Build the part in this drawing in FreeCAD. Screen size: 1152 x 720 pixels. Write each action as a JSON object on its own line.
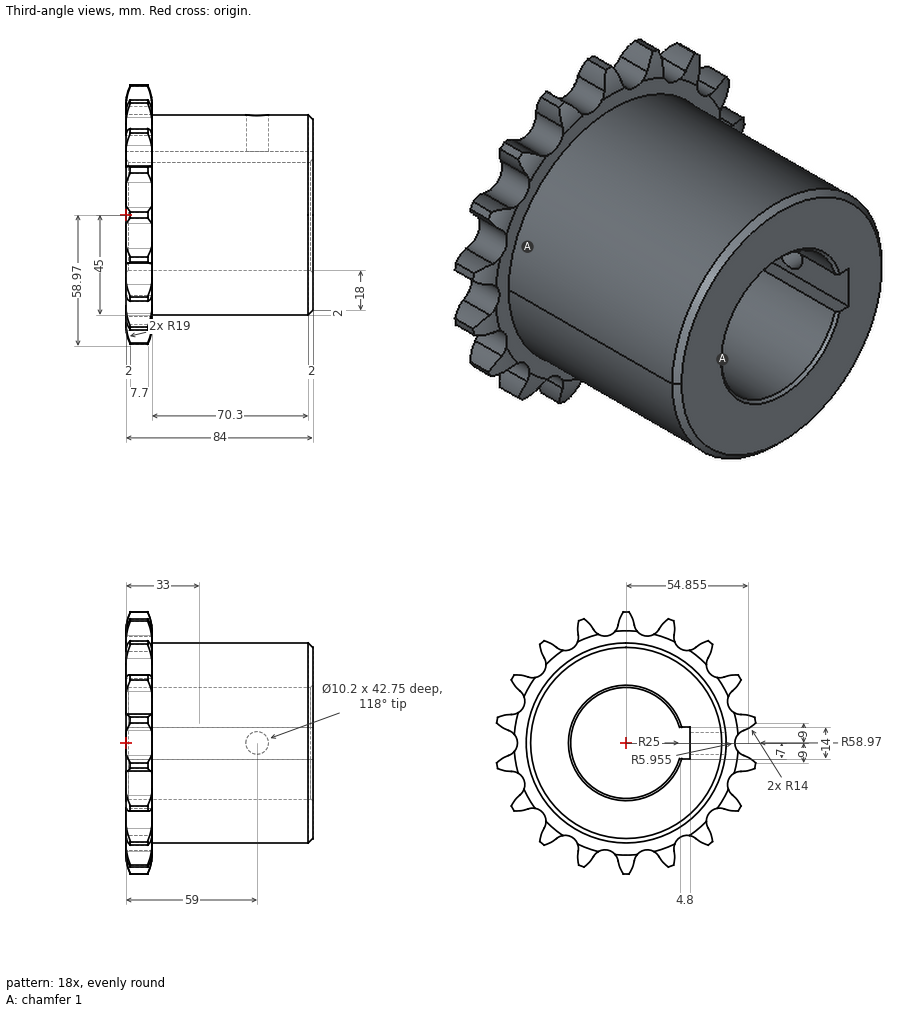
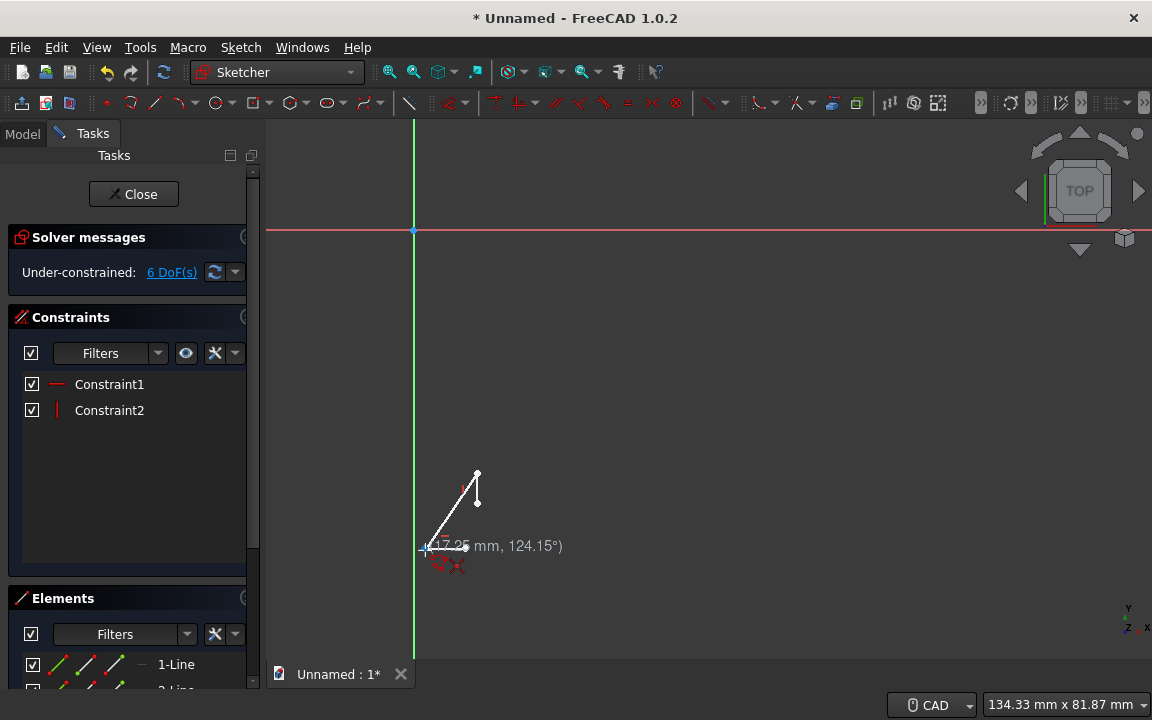
{"action": "left_click", "coordinate": [857, 473]}
{"action": "left_click", "coordinate": [868, 462]}
{"action": "left_click", "coordinate": [868, 365]}
{"action": "left_click", "coordinate": [414, 365]}
{"action": "left_click", "coordinate": [423, 503]}
{"action": "right_click", "coordinate": [423, 503]}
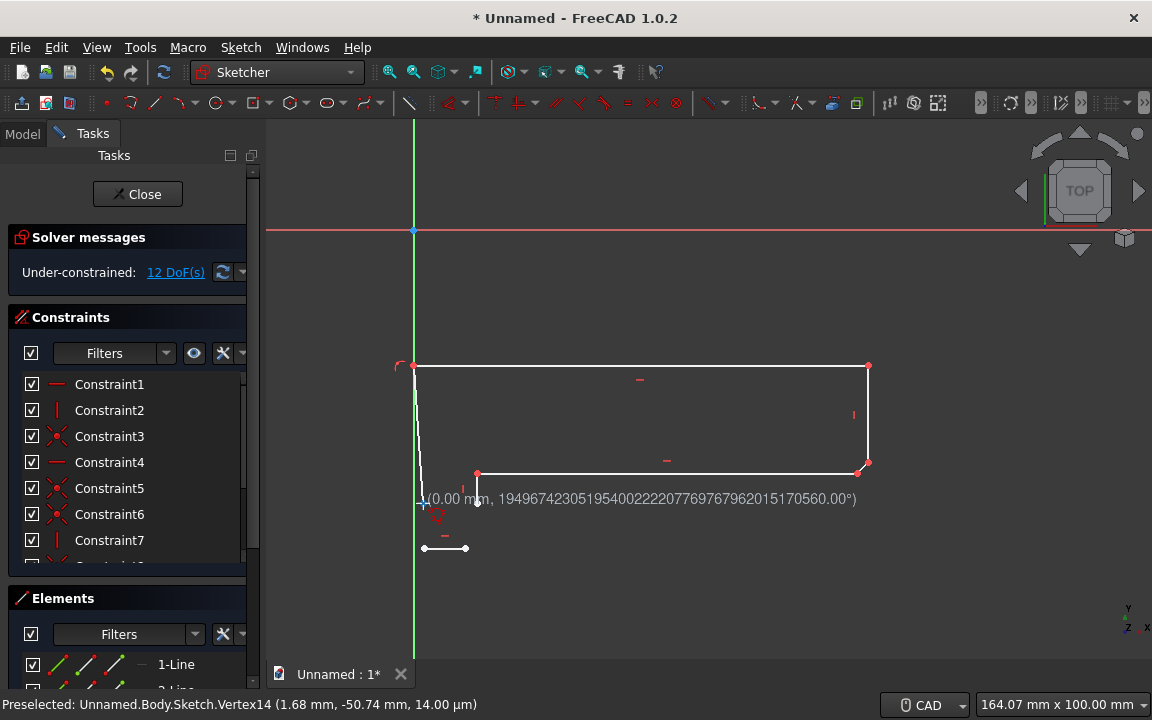
{"action": "key", "text": "g 3 a"}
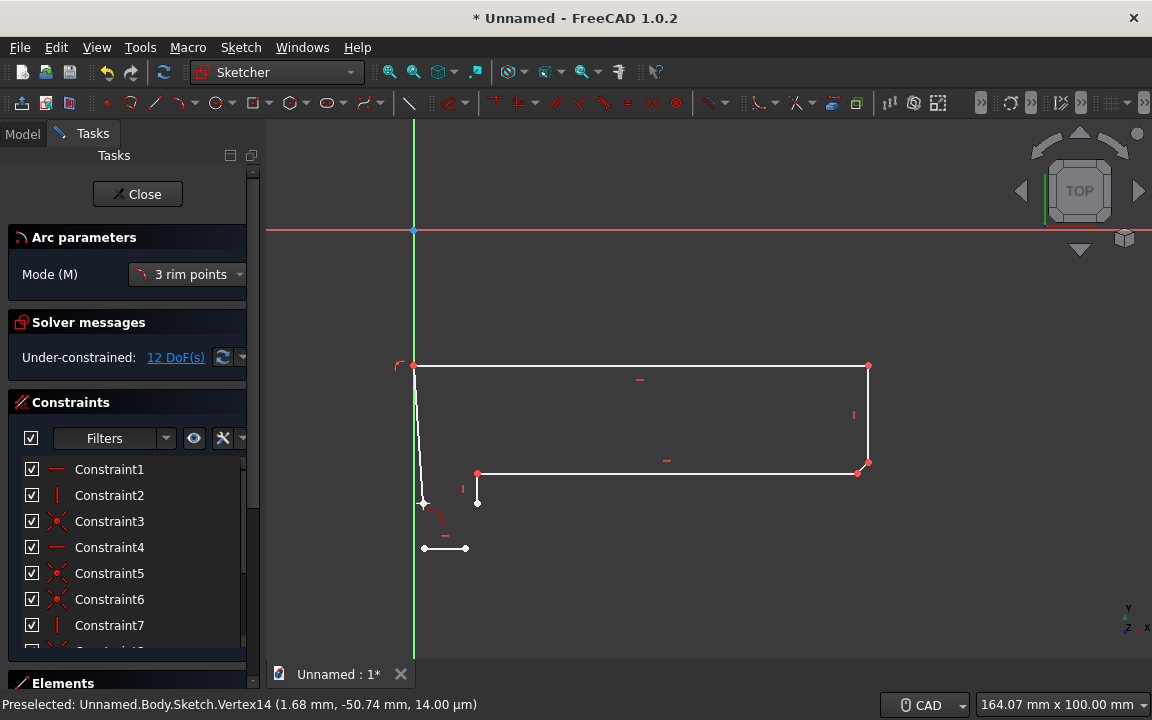
{"action": "left_click", "coordinate": [466, 549]}
{"action": "left_click", "coordinate": [477, 503]}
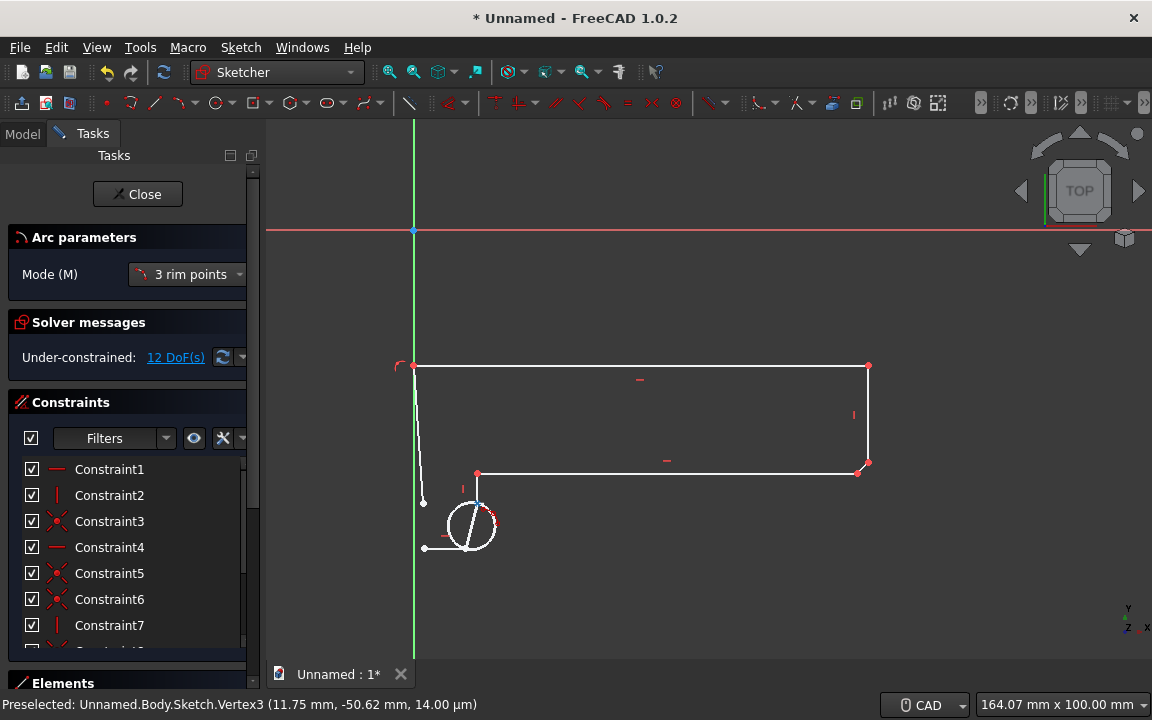
{"action": "scroll", "coordinate": [474, 526], "scroll_direction": "up", "scroll_amount": 9}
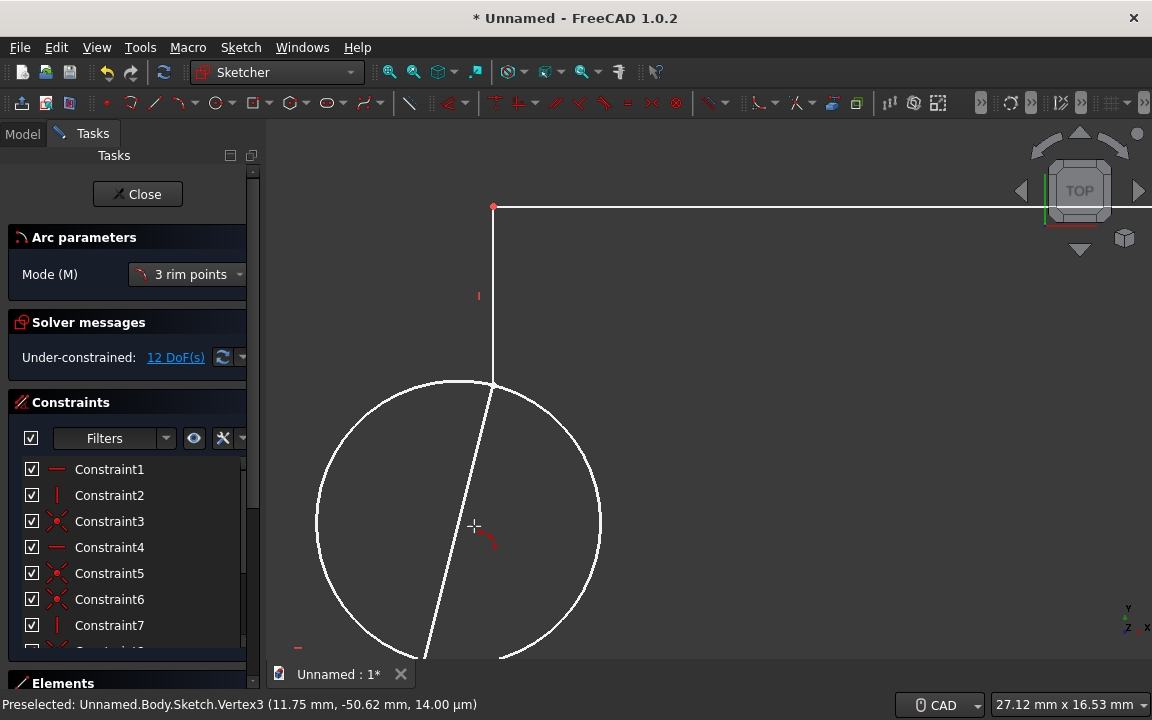
{"action": "left_click", "coordinate": [475, 523]}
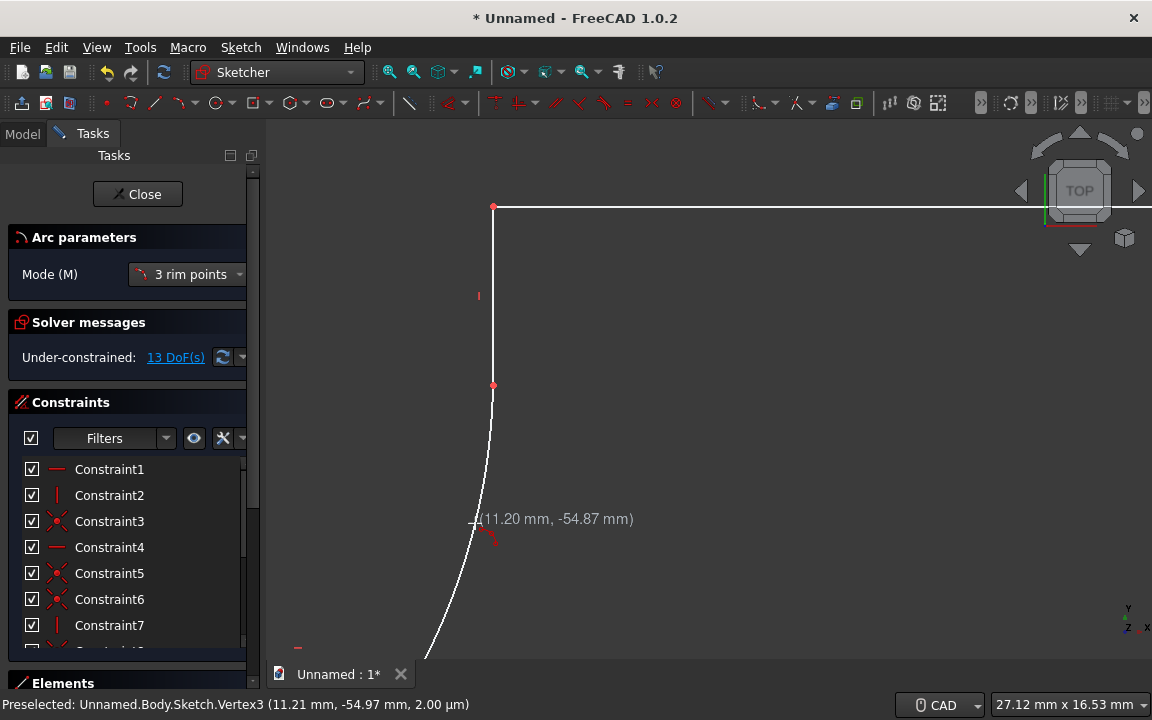
{"action": "scroll", "coordinate": [474, 526], "scroll_direction": "down", "scroll_amount": 9}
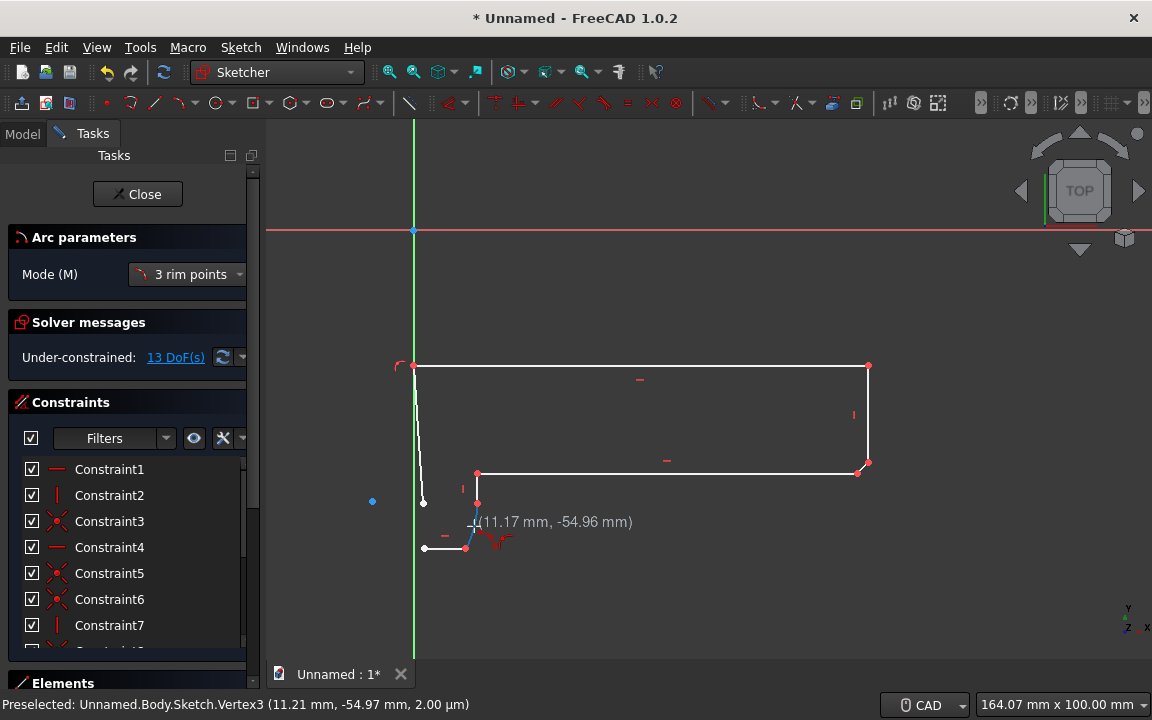
{"action": "left_click", "coordinate": [423, 504]}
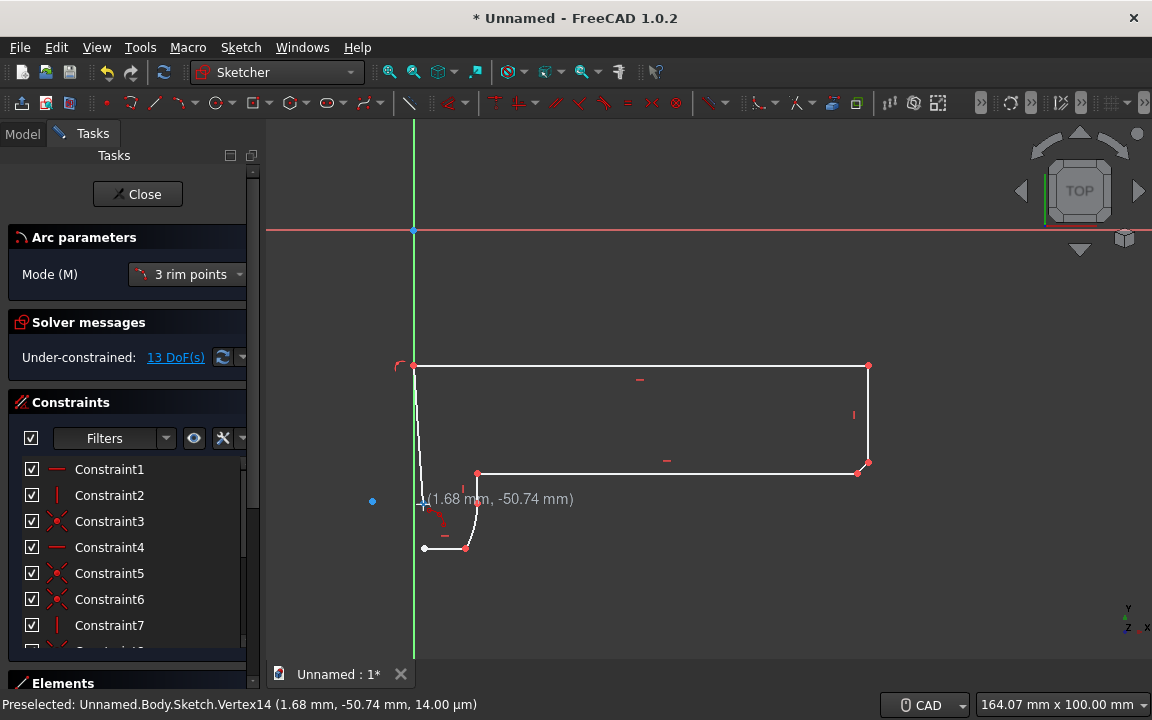
{"action": "scroll", "coordinate": [425, 548], "scroll_direction": "up", "scroll_amount": 2}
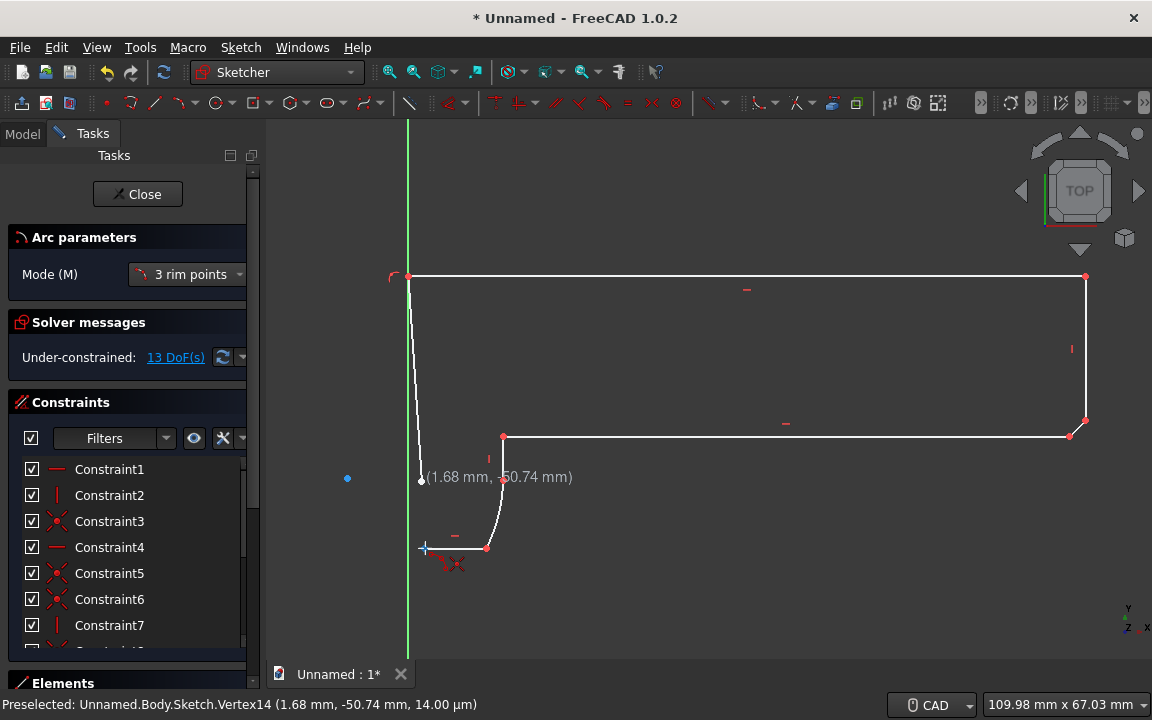
{"action": "left_click", "coordinate": [424, 549]}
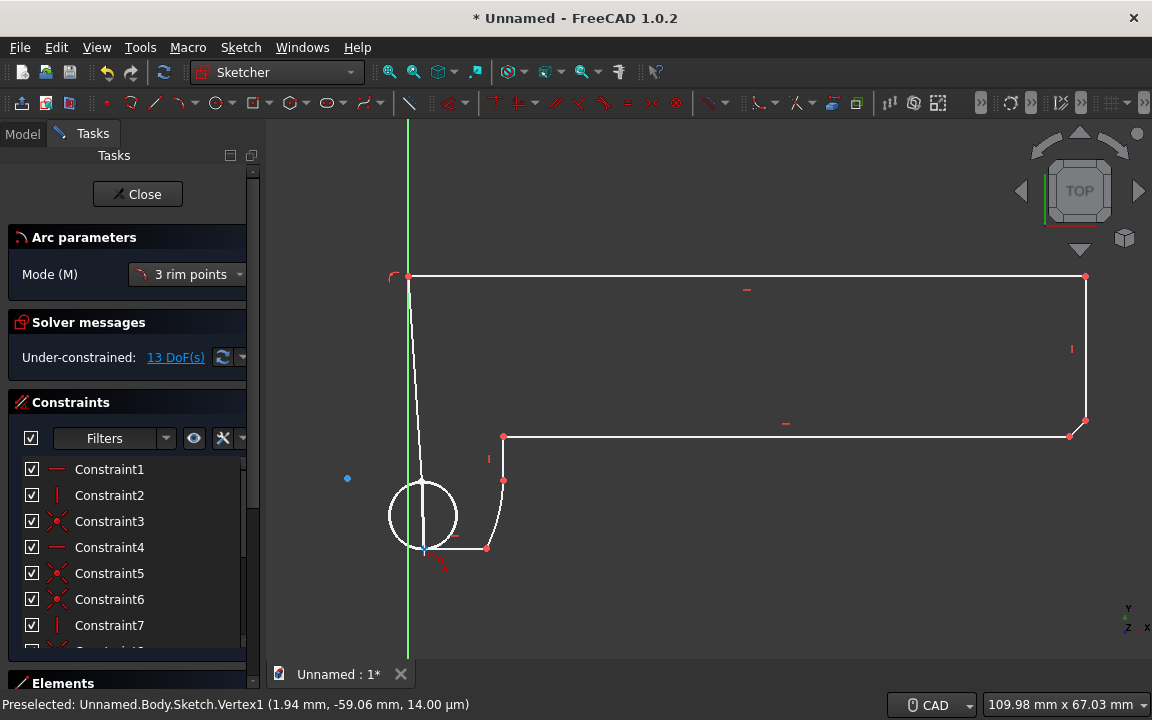
{"action": "scroll", "coordinate": [412, 515], "scroll_direction": "up", "scroll_amount": 7}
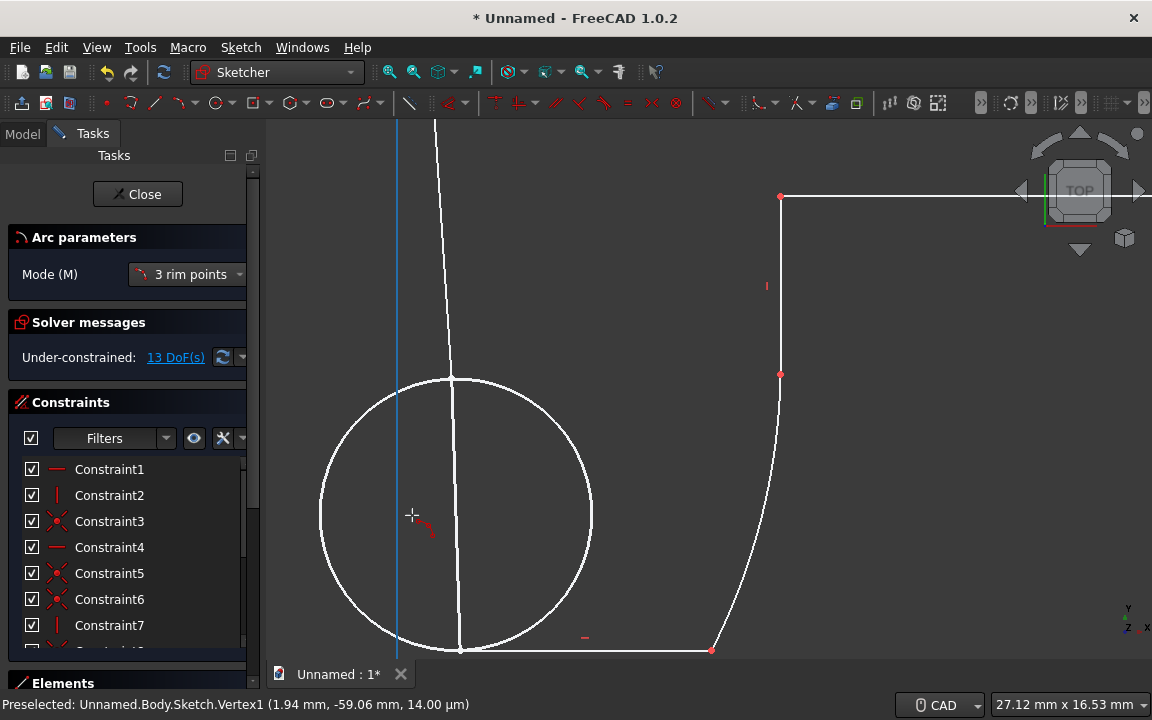
{"action": "left_click", "coordinate": [413, 513]}
{"action": "key", "text": "Escape"}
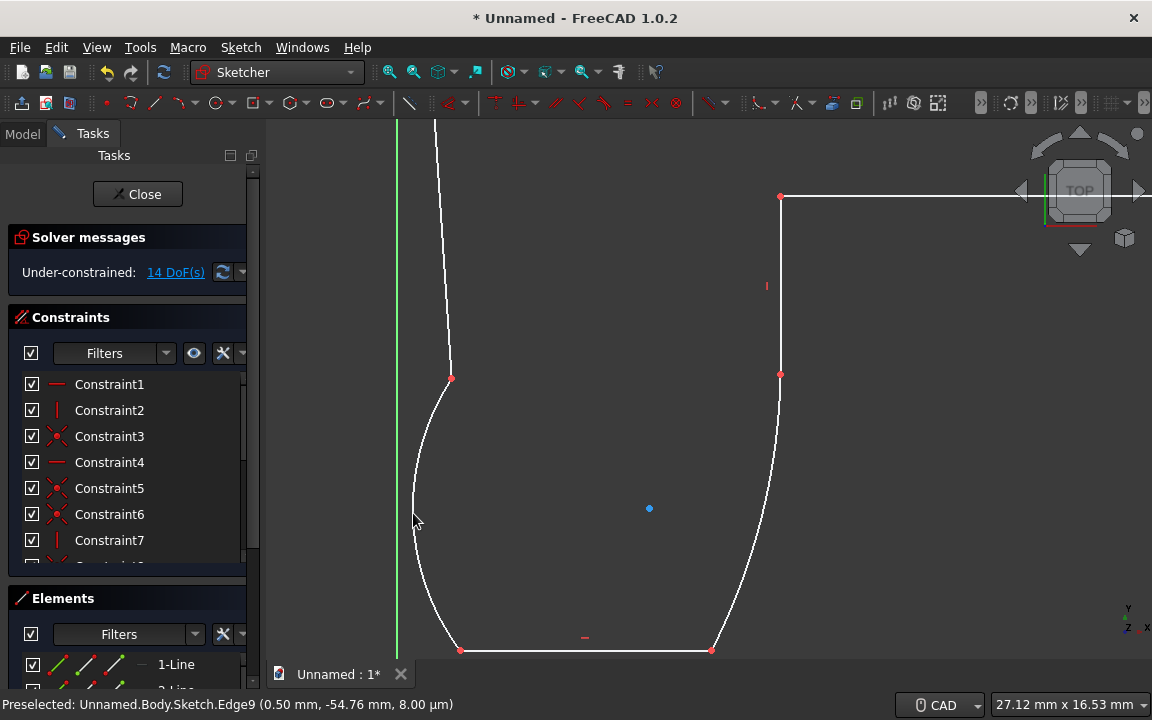
{"action": "scroll", "coordinate": [417, 529], "scroll_direction": "down", "scroll_amount": 9}